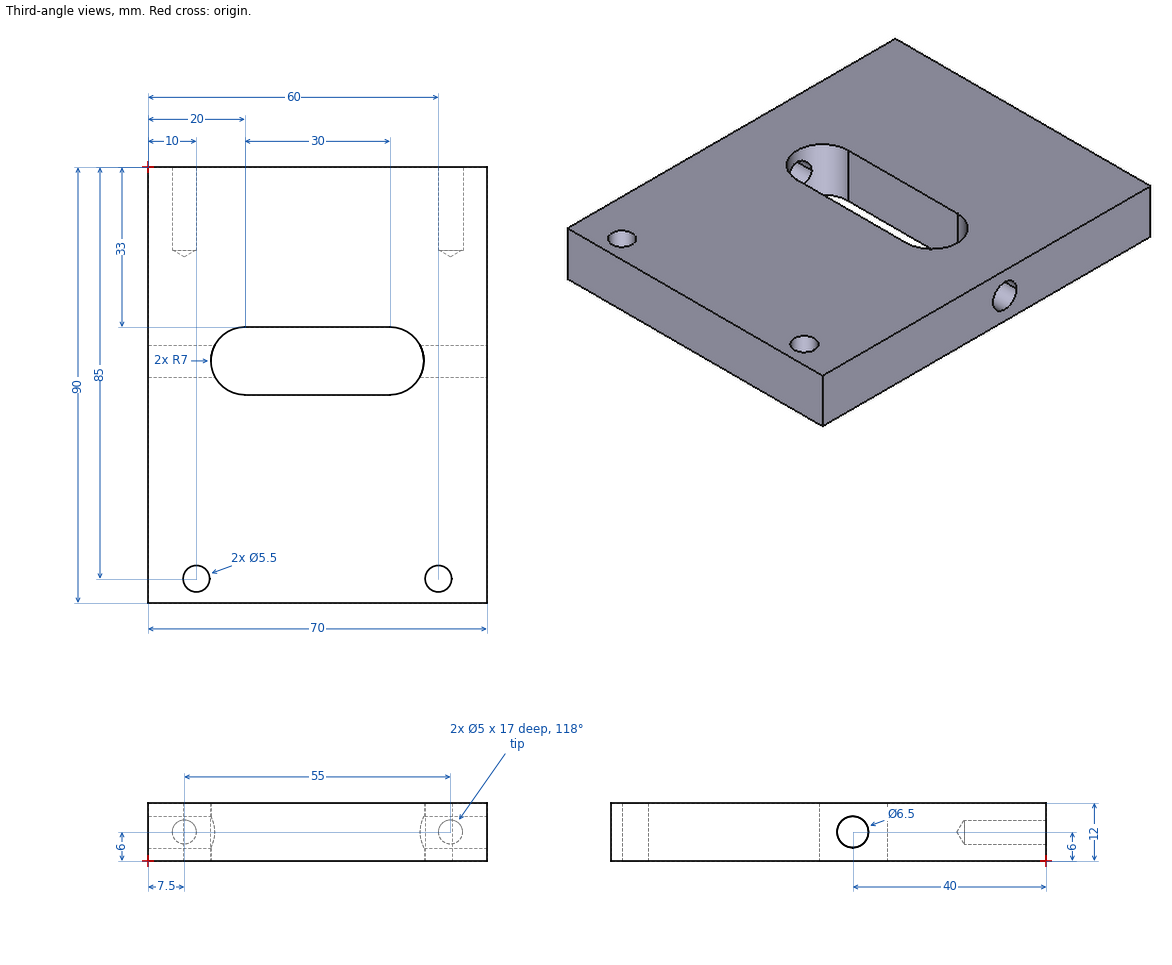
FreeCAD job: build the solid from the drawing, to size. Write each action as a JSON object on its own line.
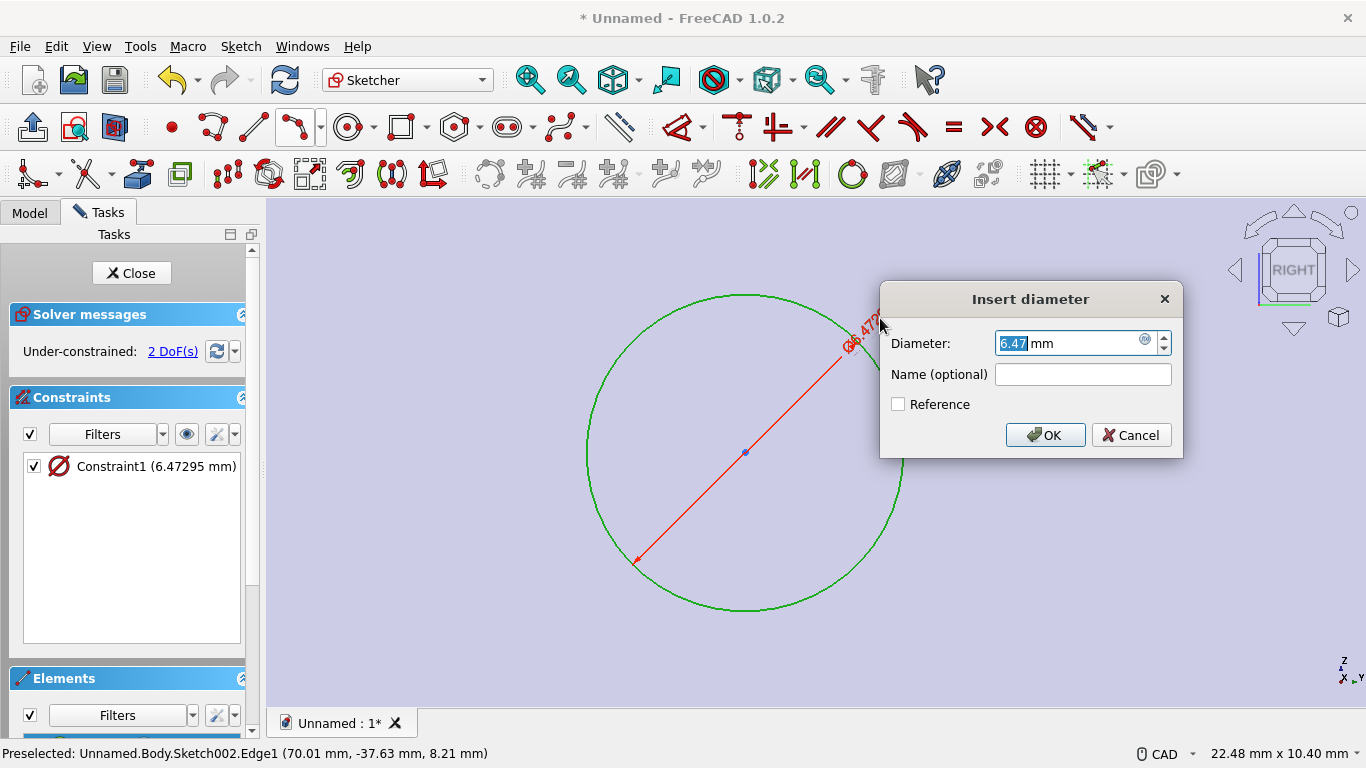
{"action": "type", "text": "6.5"}
{"action": "key", "text": "Return"}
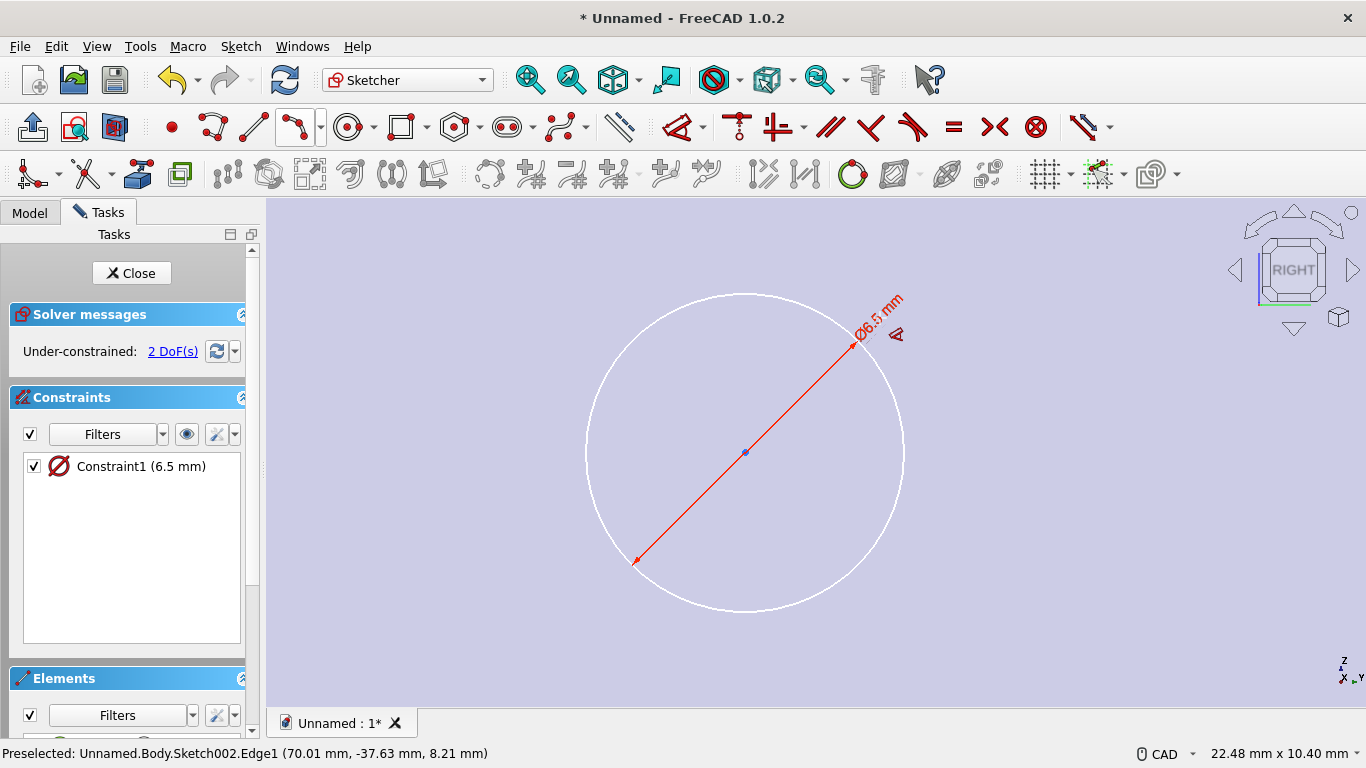
{"action": "left_click", "coordinate": [745, 453]}
{"action": "left_click", "coordinate": [711, 566]}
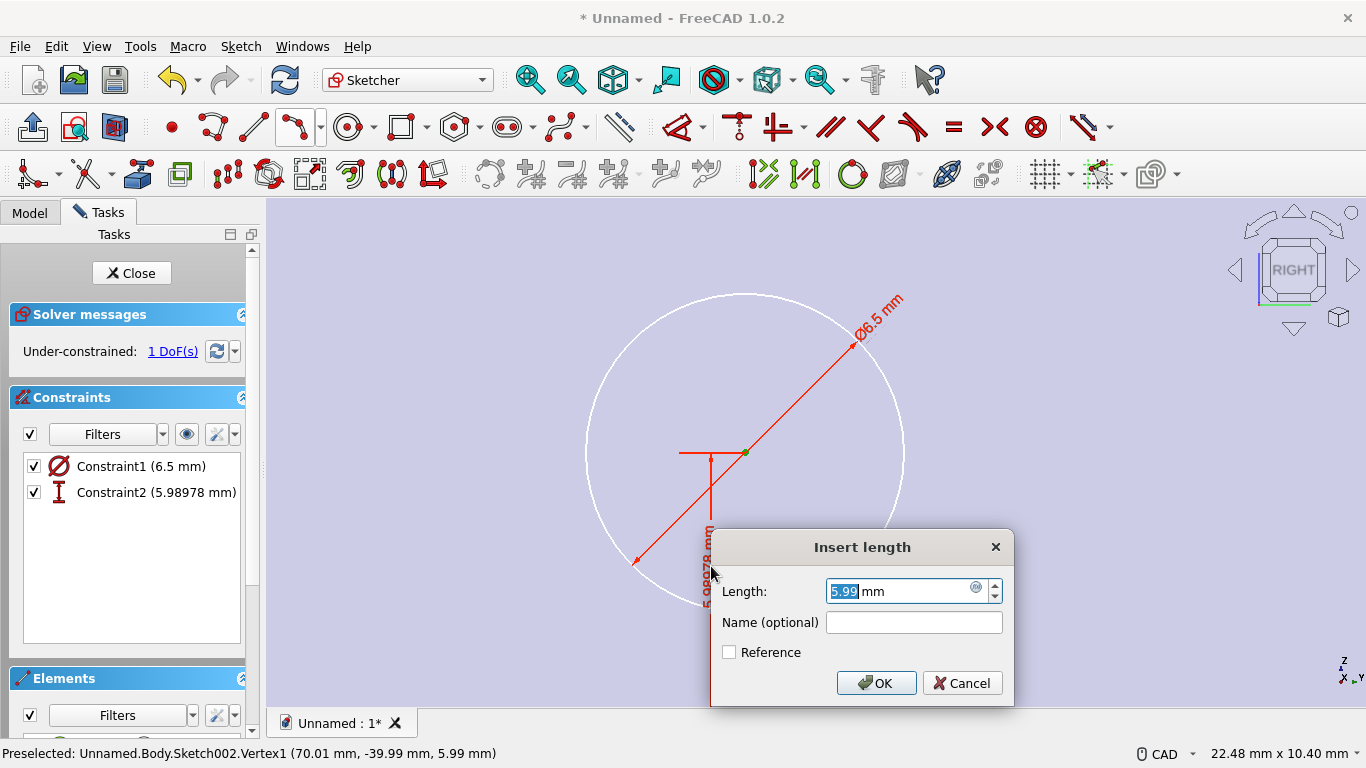
{"action": "type", "text": "6"}
{"action": "key", "text": "Return"}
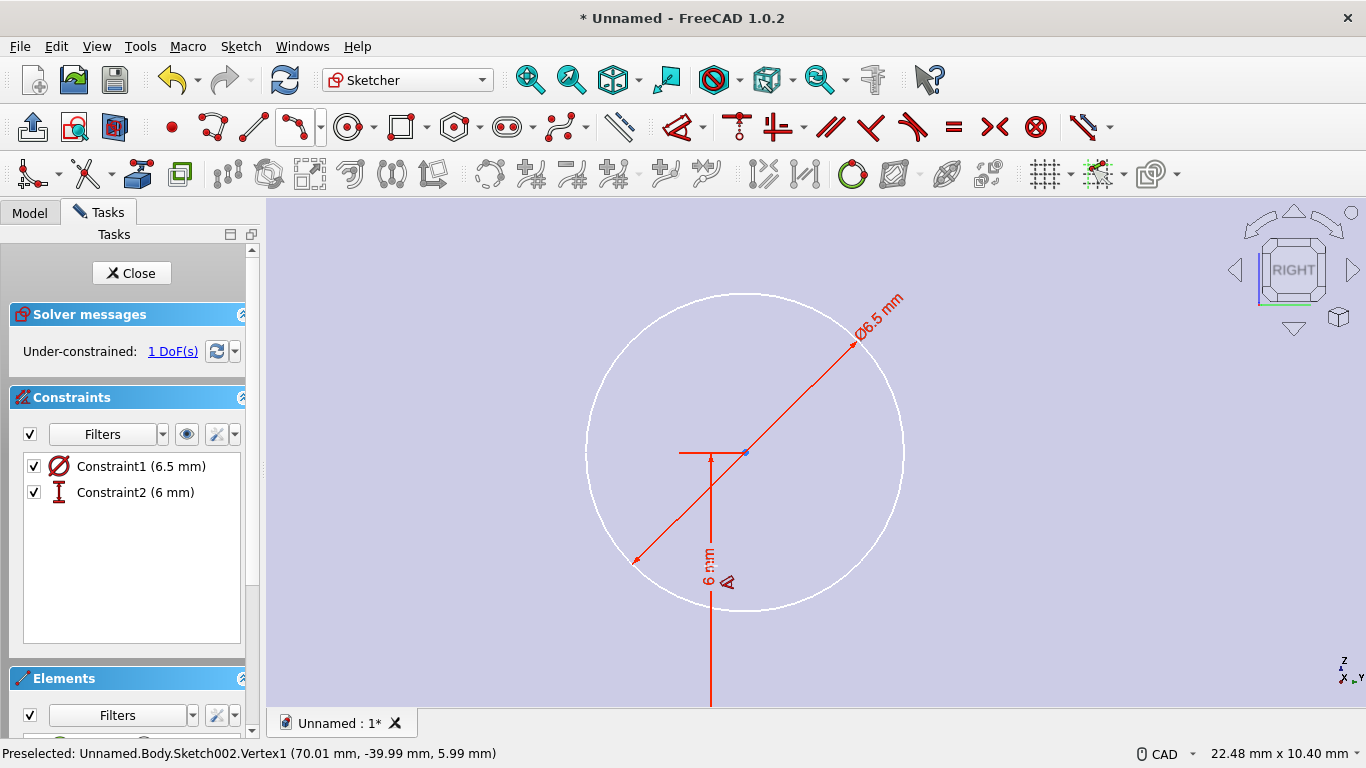
{"action": "left_click", "coordinate": [745, 452]}
{"action": "left_click", "coordinate": [973, 418]}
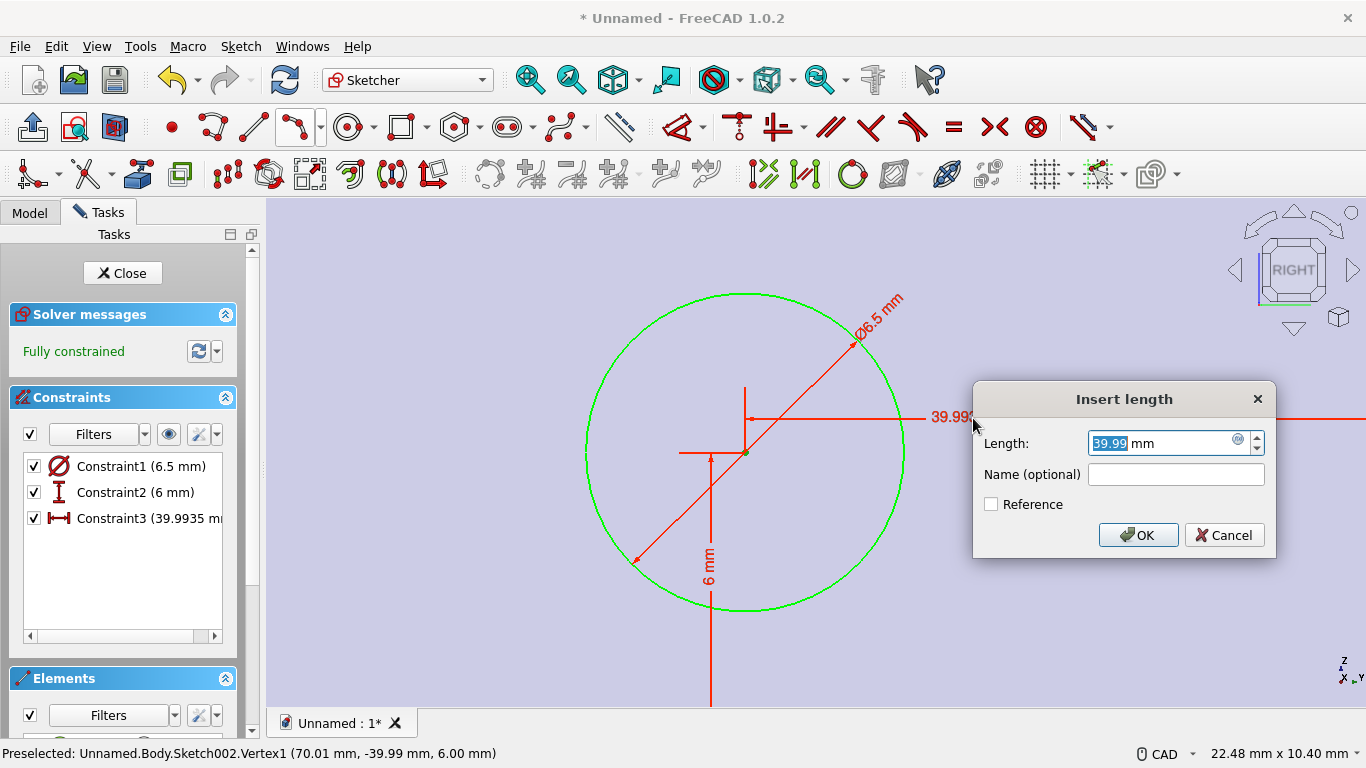
{"action": "type", "text": "40"}
{"action": "key", "text": "Return"}
{"action": "key", "text": "Escape"}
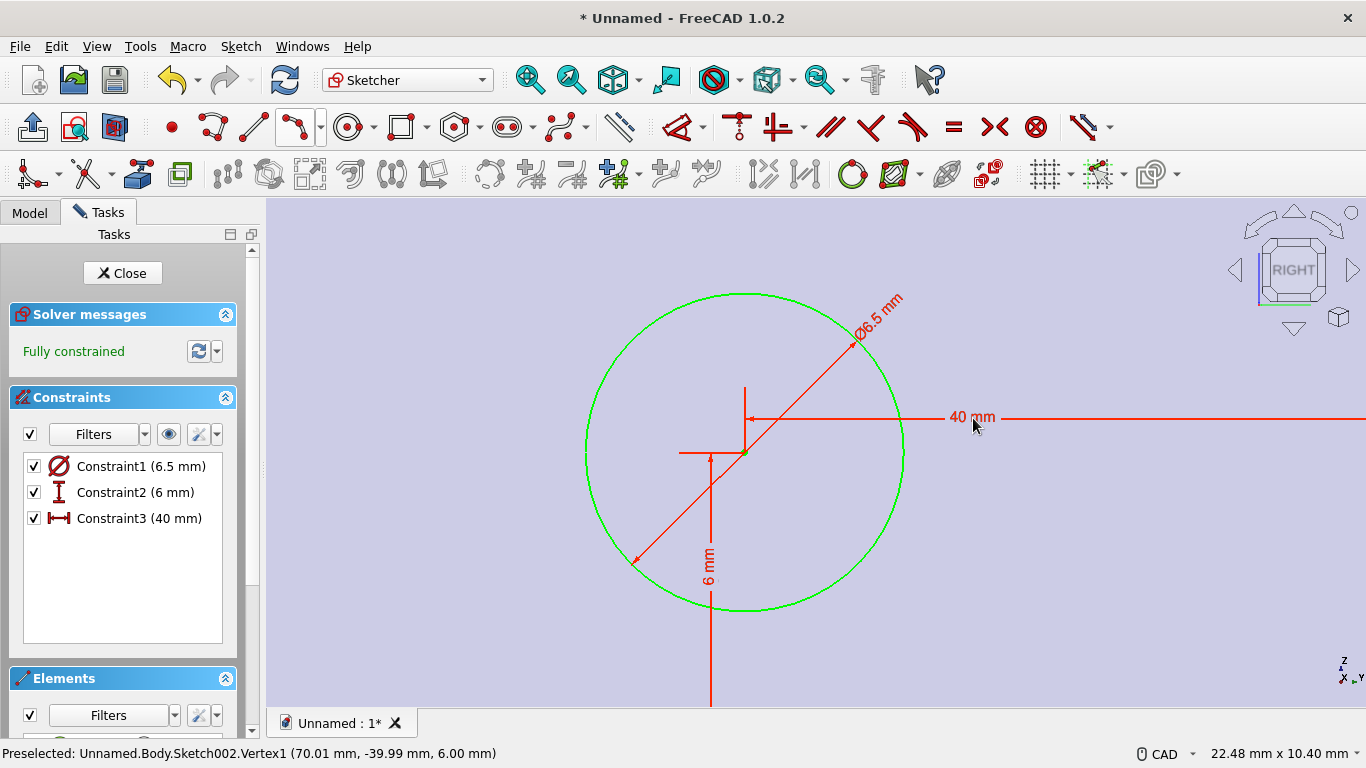
{"action": "left_click", "coordinate": [123, 273]}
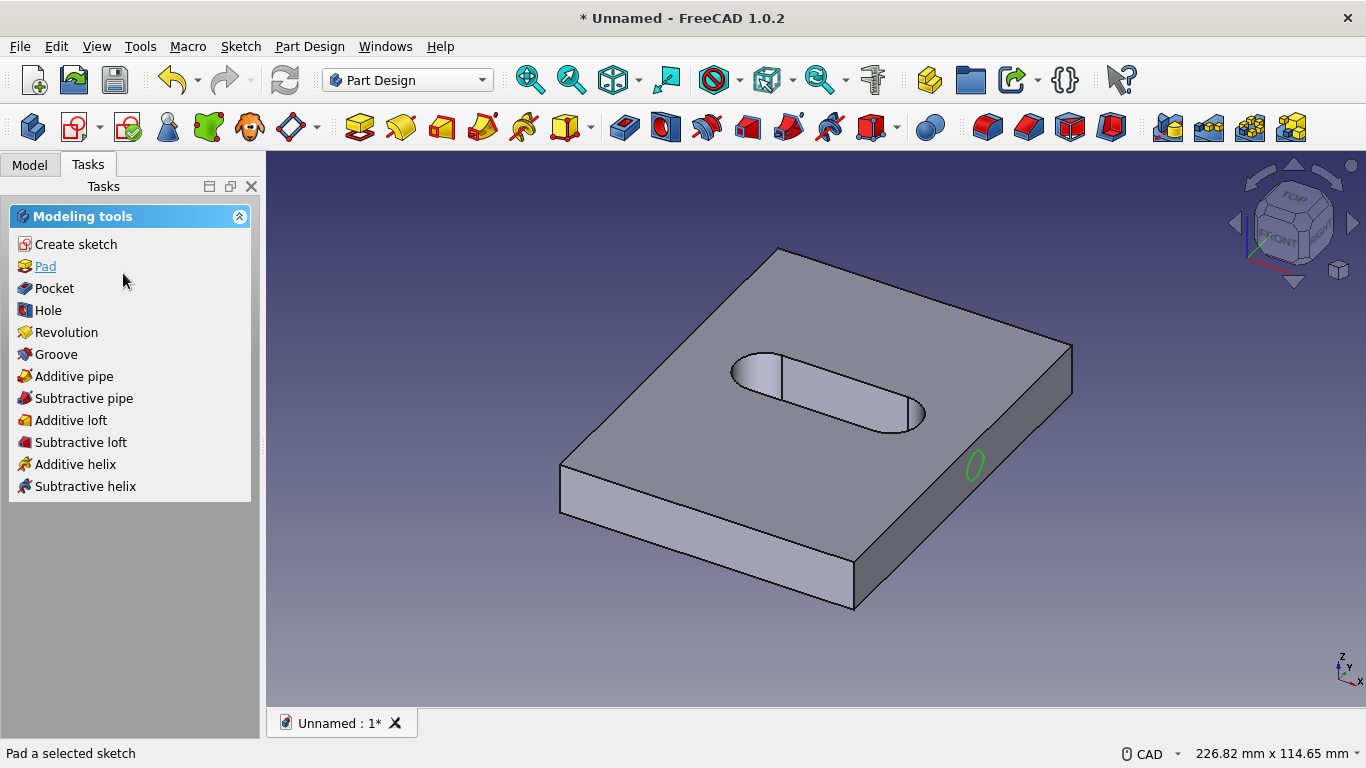
{"action": "left_click", "coordinate": [625, 128]}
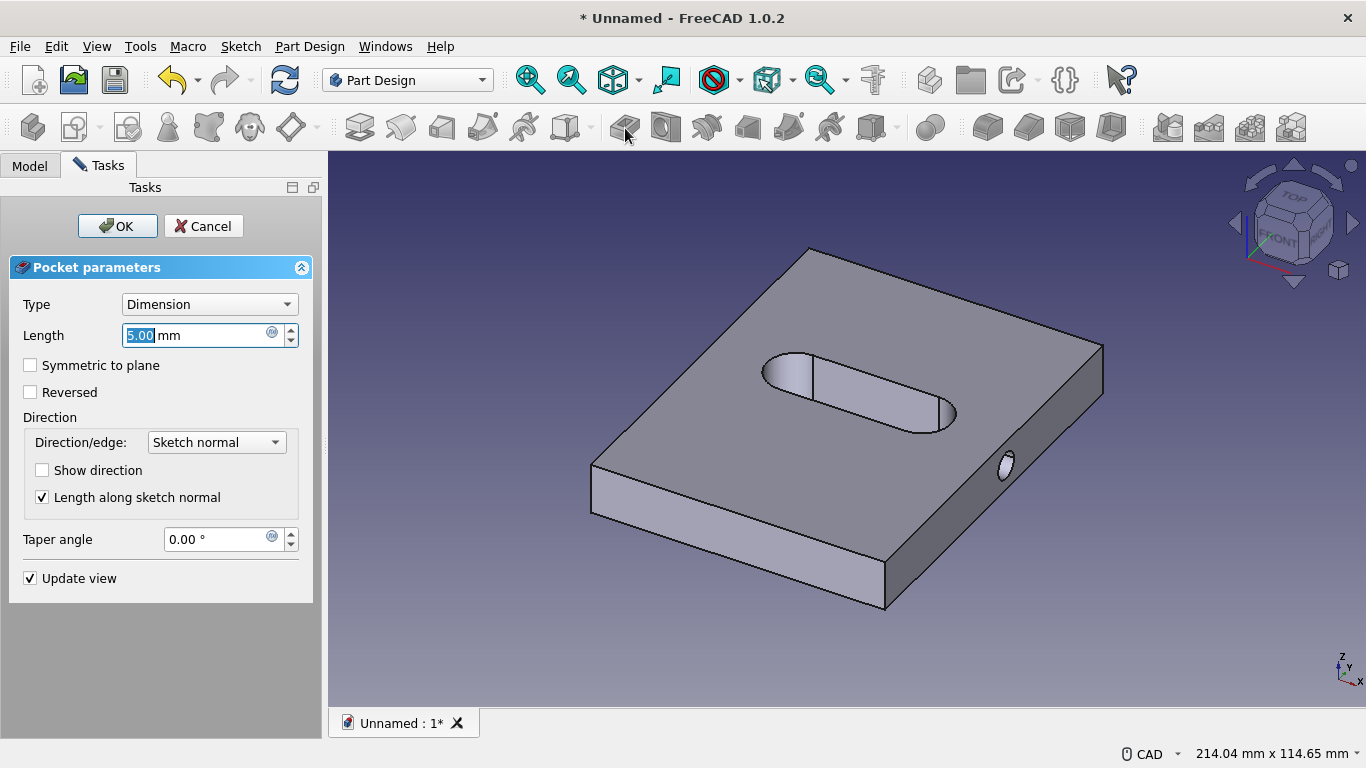
{"action": "left_click", "coordinate": [210, 304]}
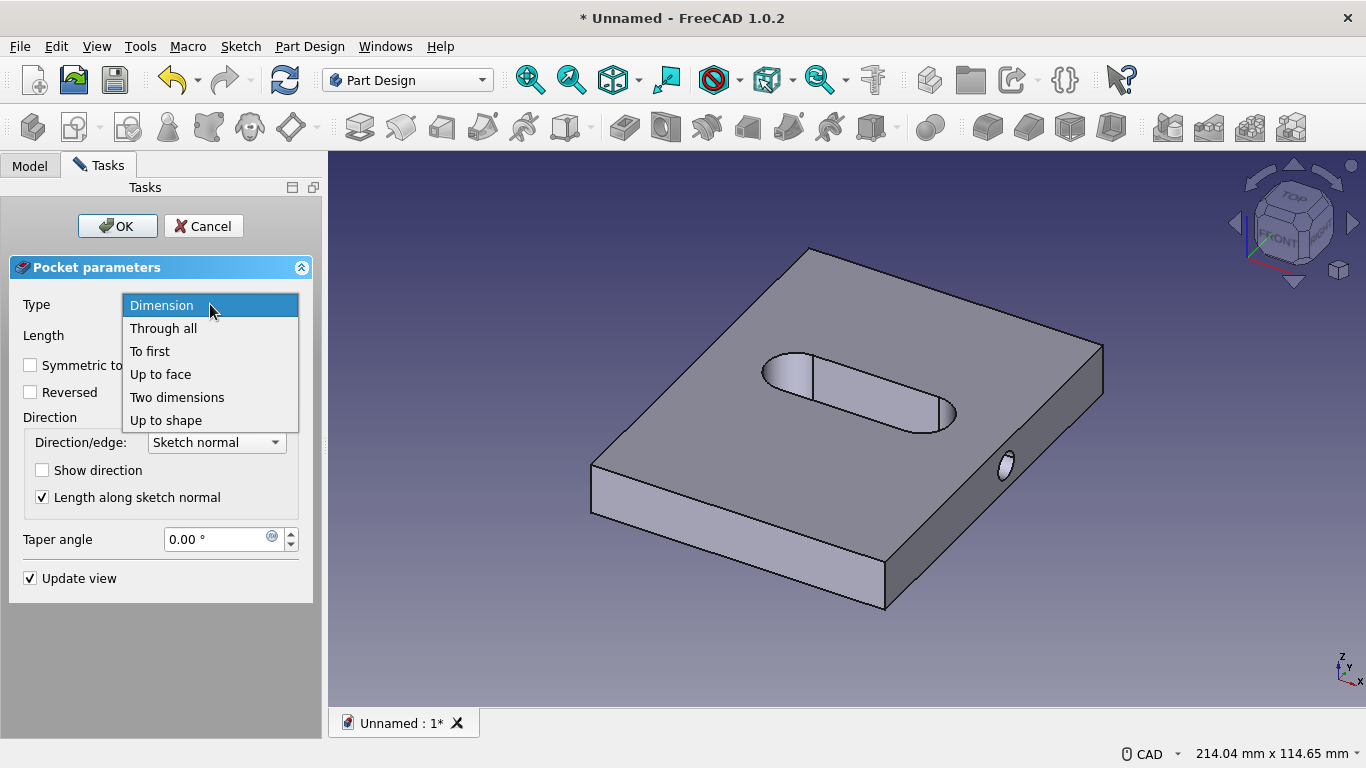
{"action": "left_click", "coordinate": [208, 328]}